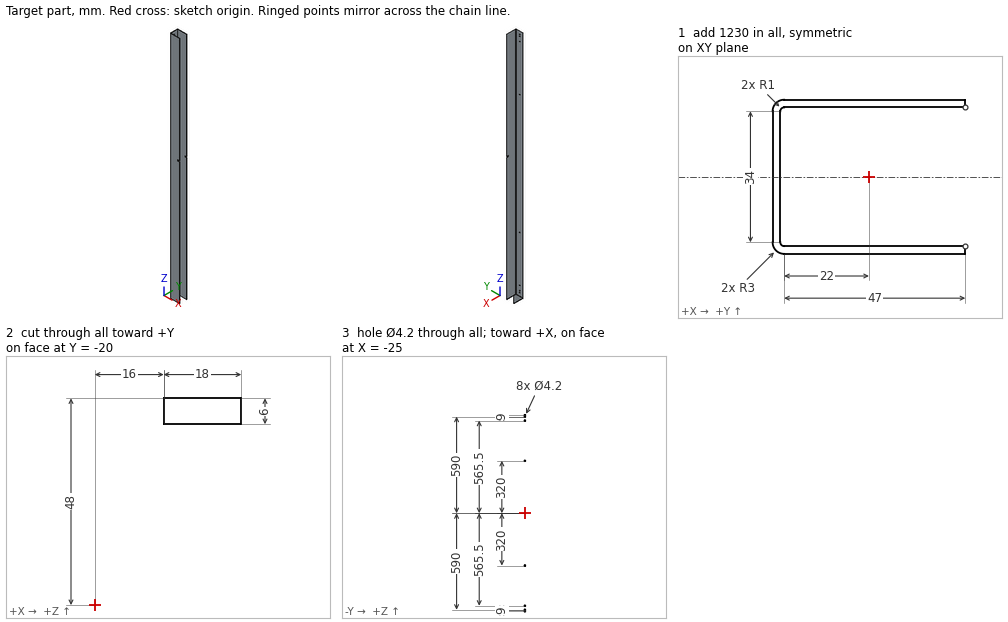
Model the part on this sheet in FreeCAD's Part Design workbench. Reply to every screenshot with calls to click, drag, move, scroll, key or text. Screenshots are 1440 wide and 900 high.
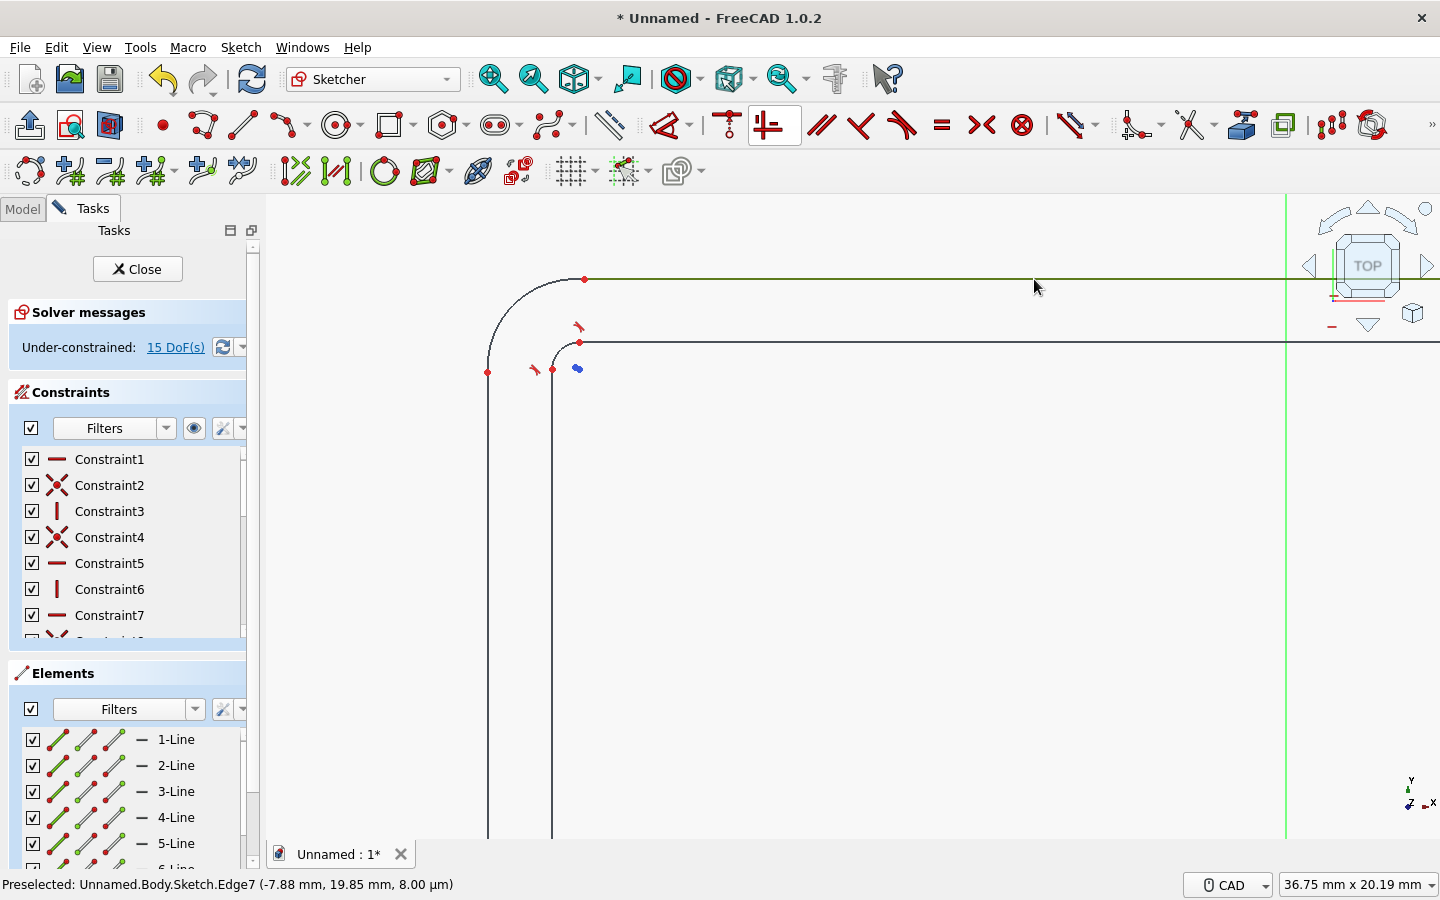
click(540, 287)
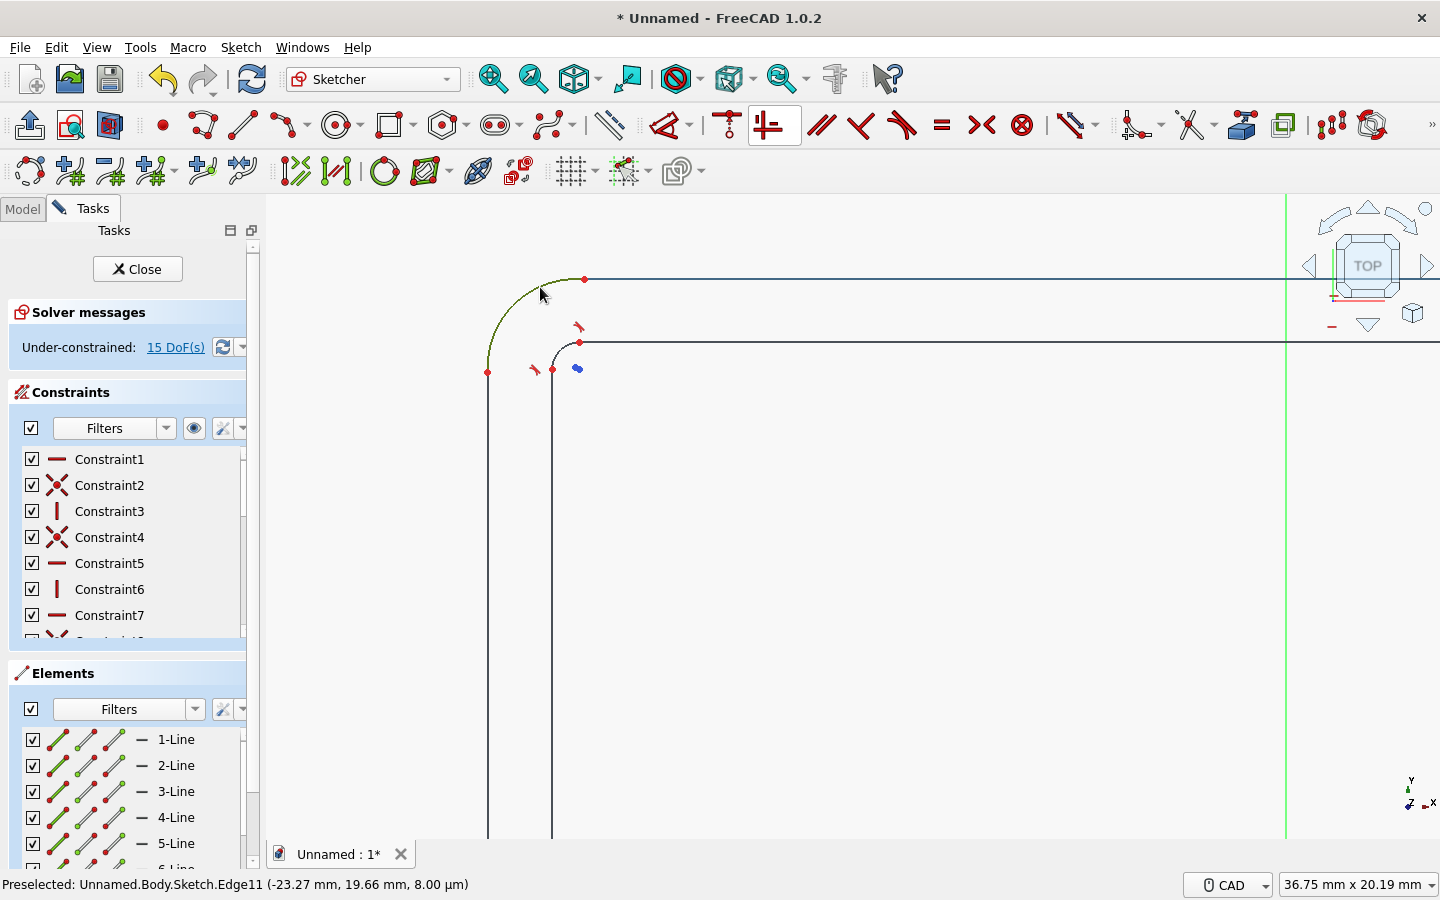
click(902, 126)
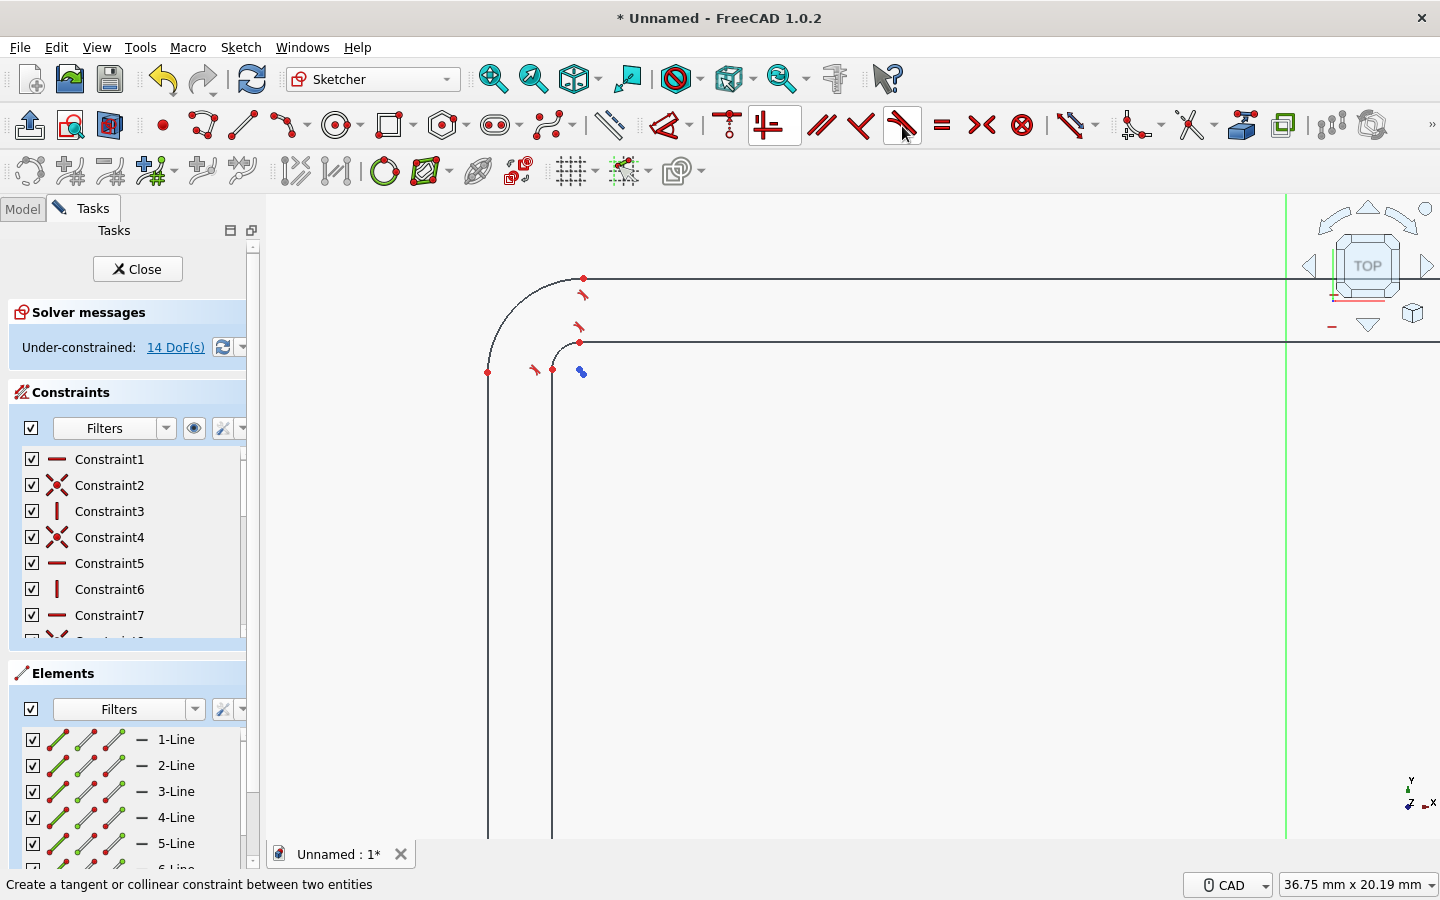
click(488, 699)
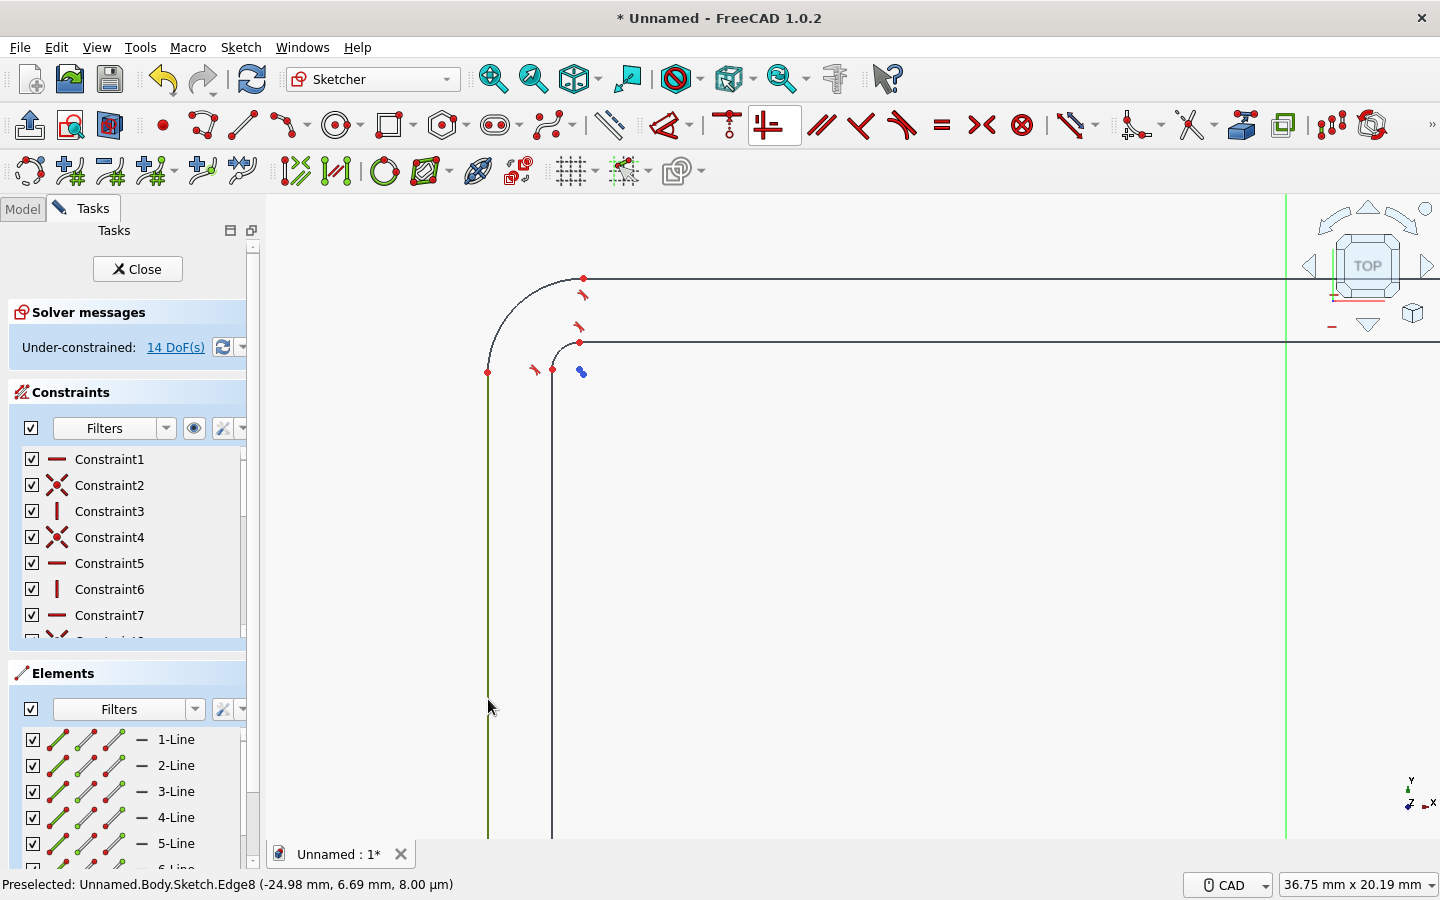
click(541, 289)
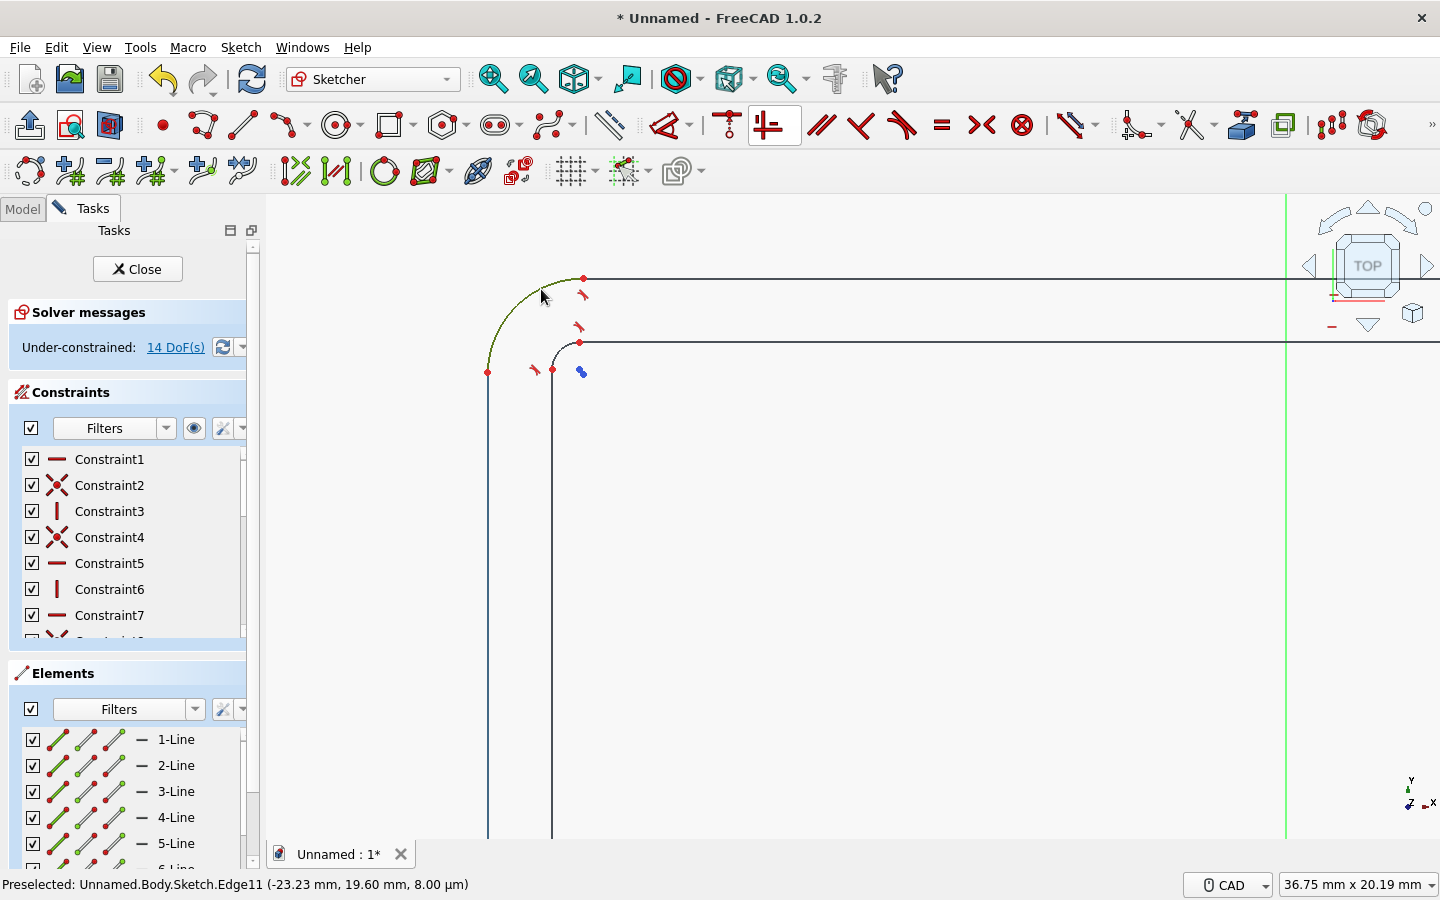
key(t)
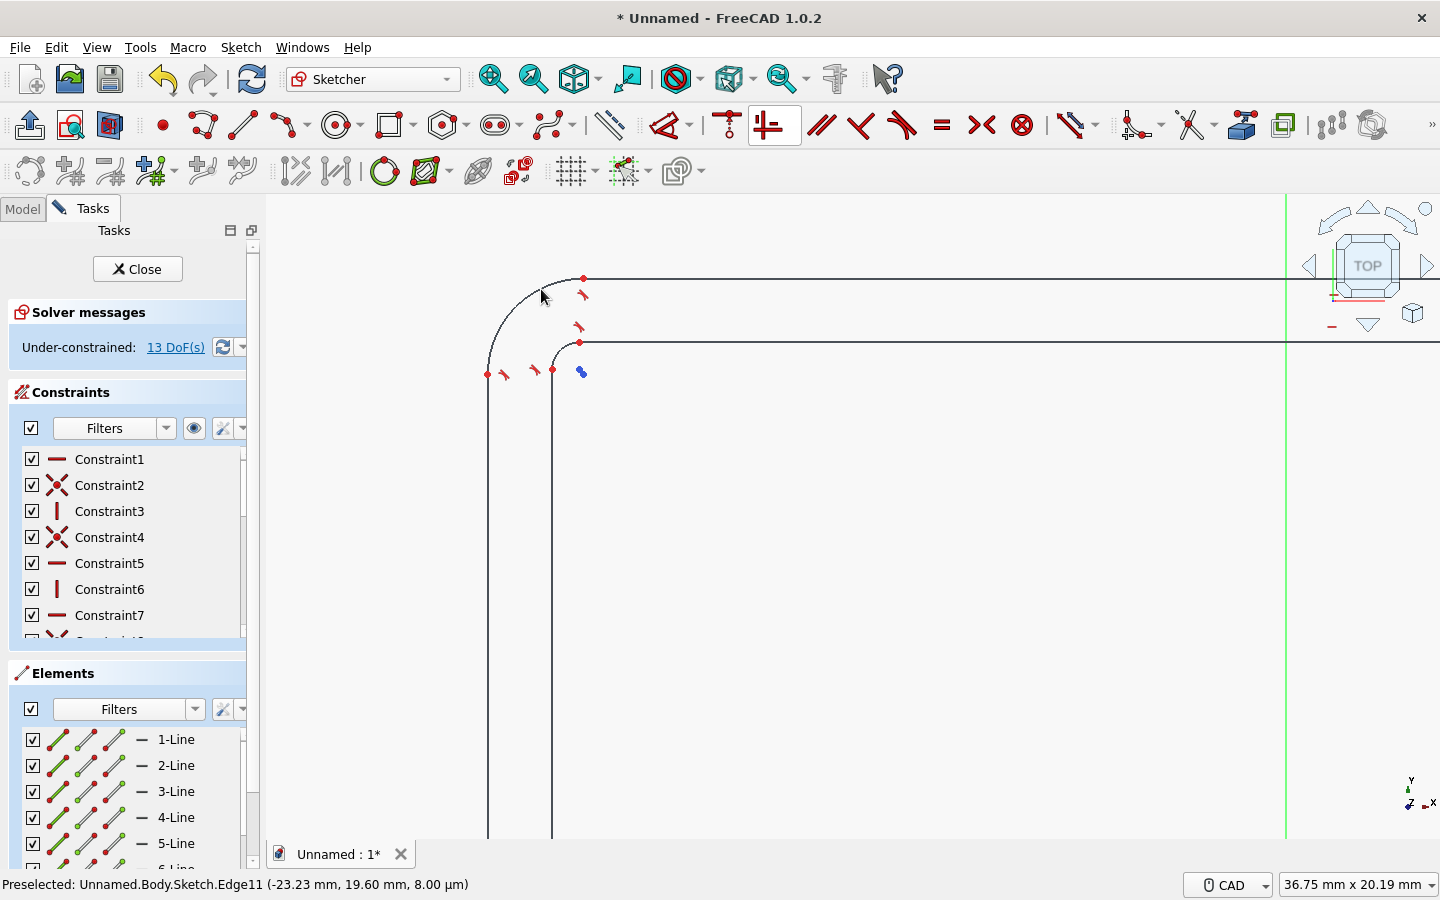
click(488, 701)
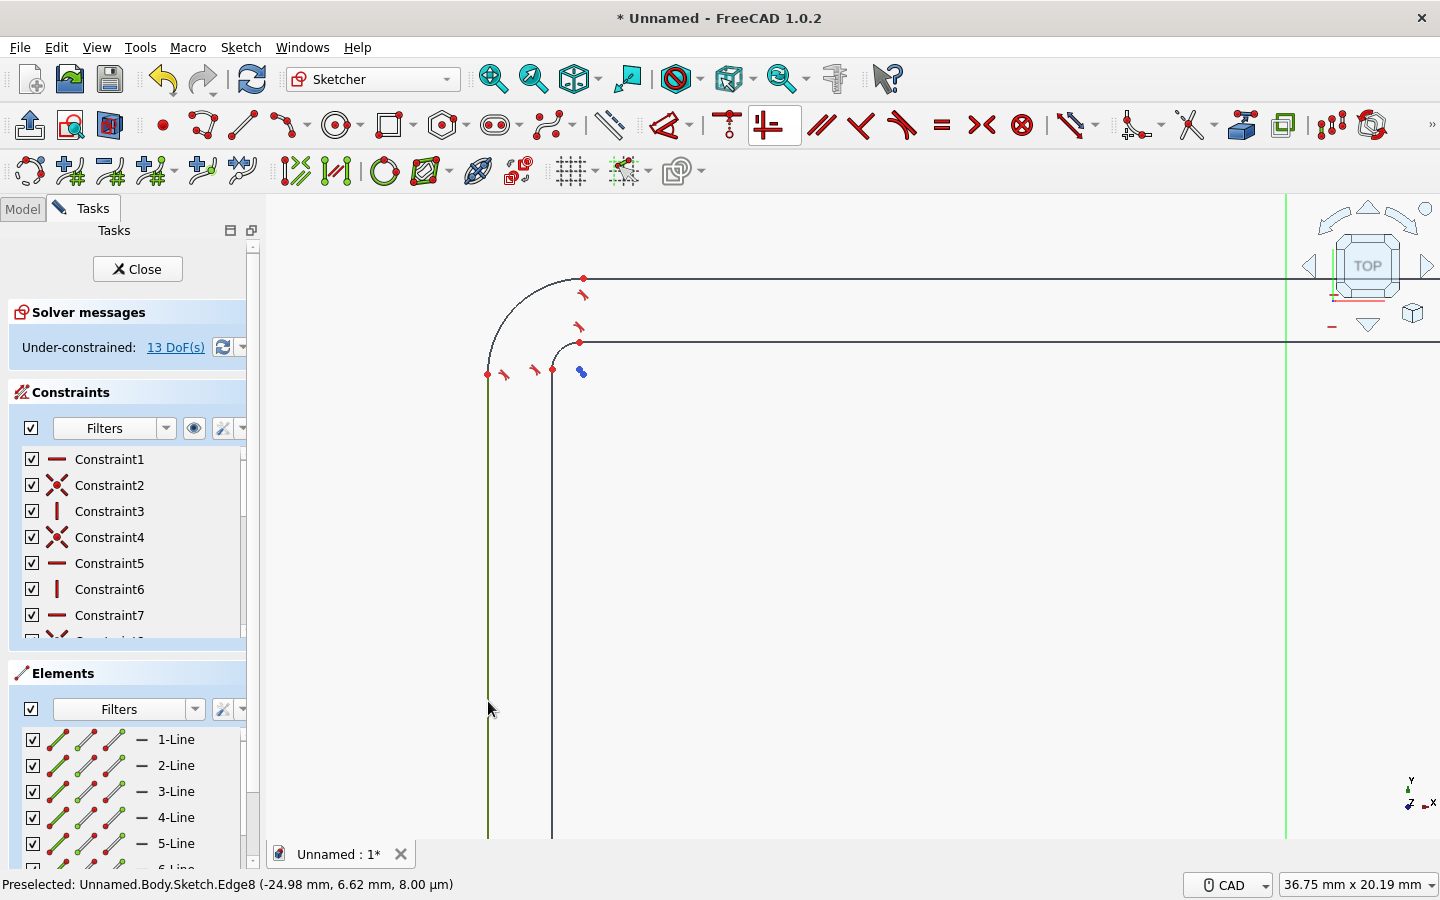
scroll(568, 345, down, 6)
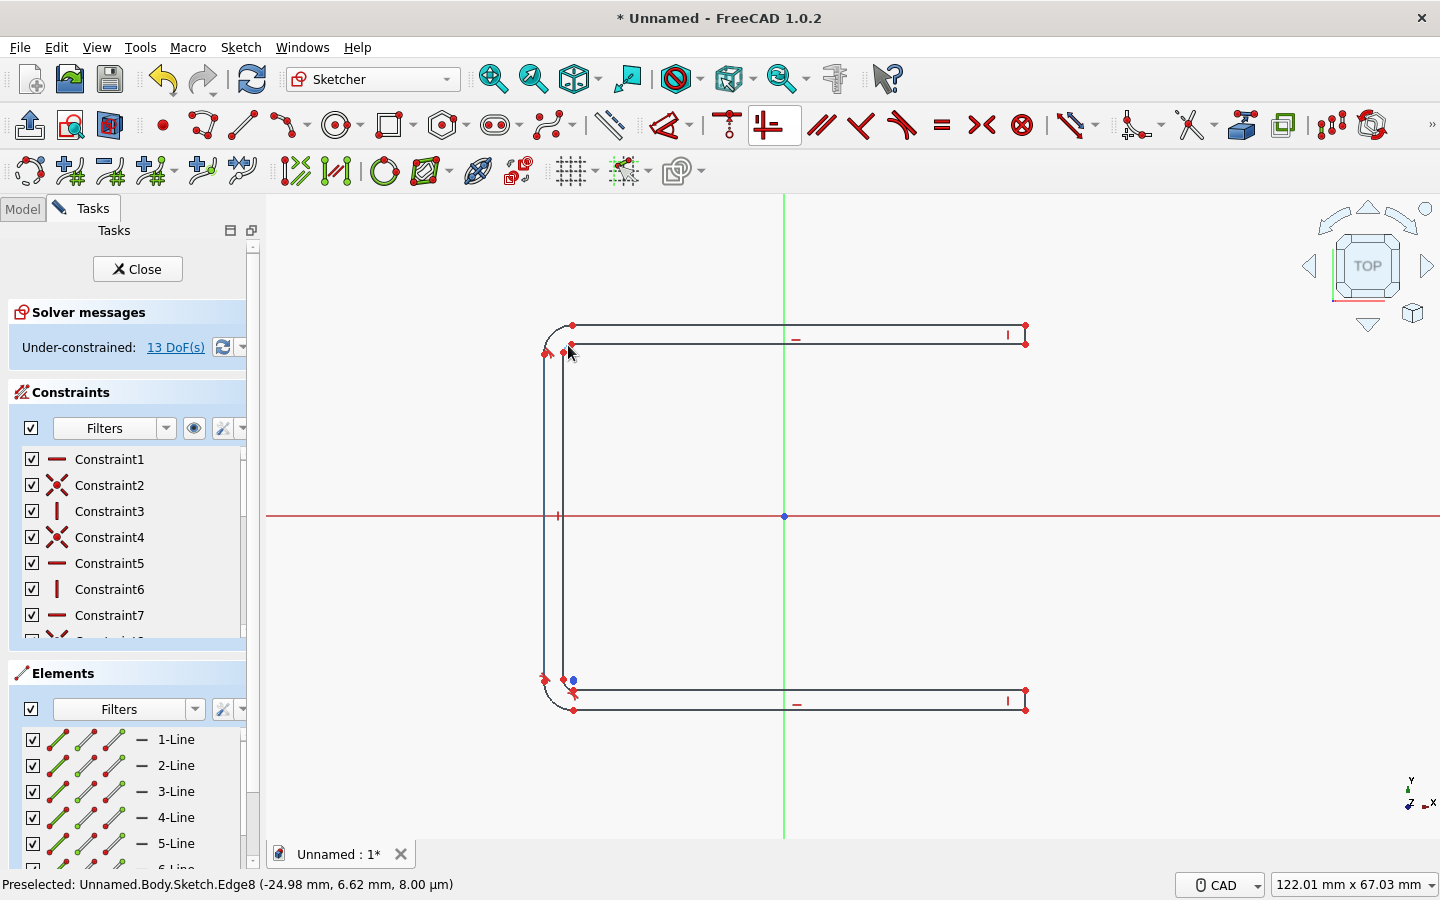
click(547, 694)